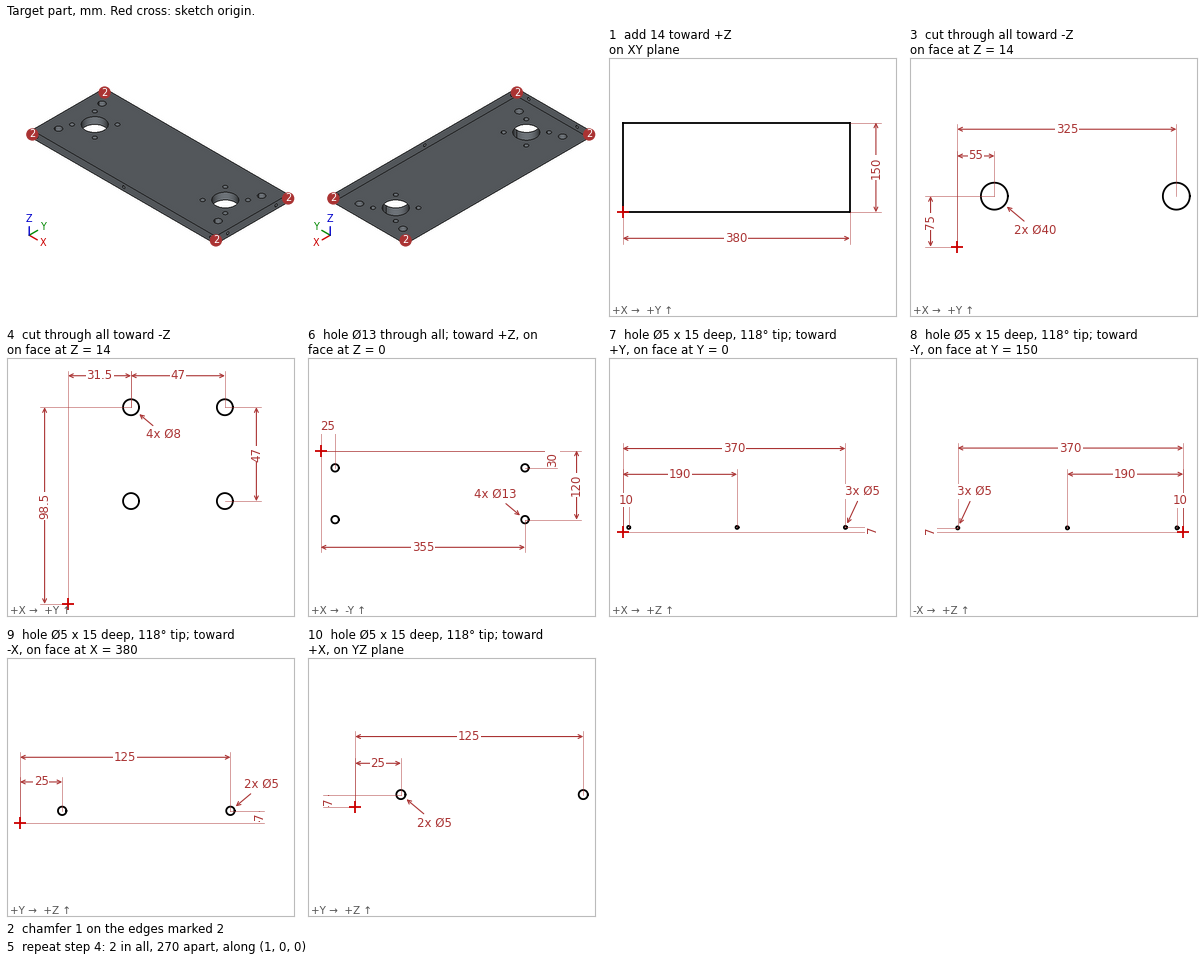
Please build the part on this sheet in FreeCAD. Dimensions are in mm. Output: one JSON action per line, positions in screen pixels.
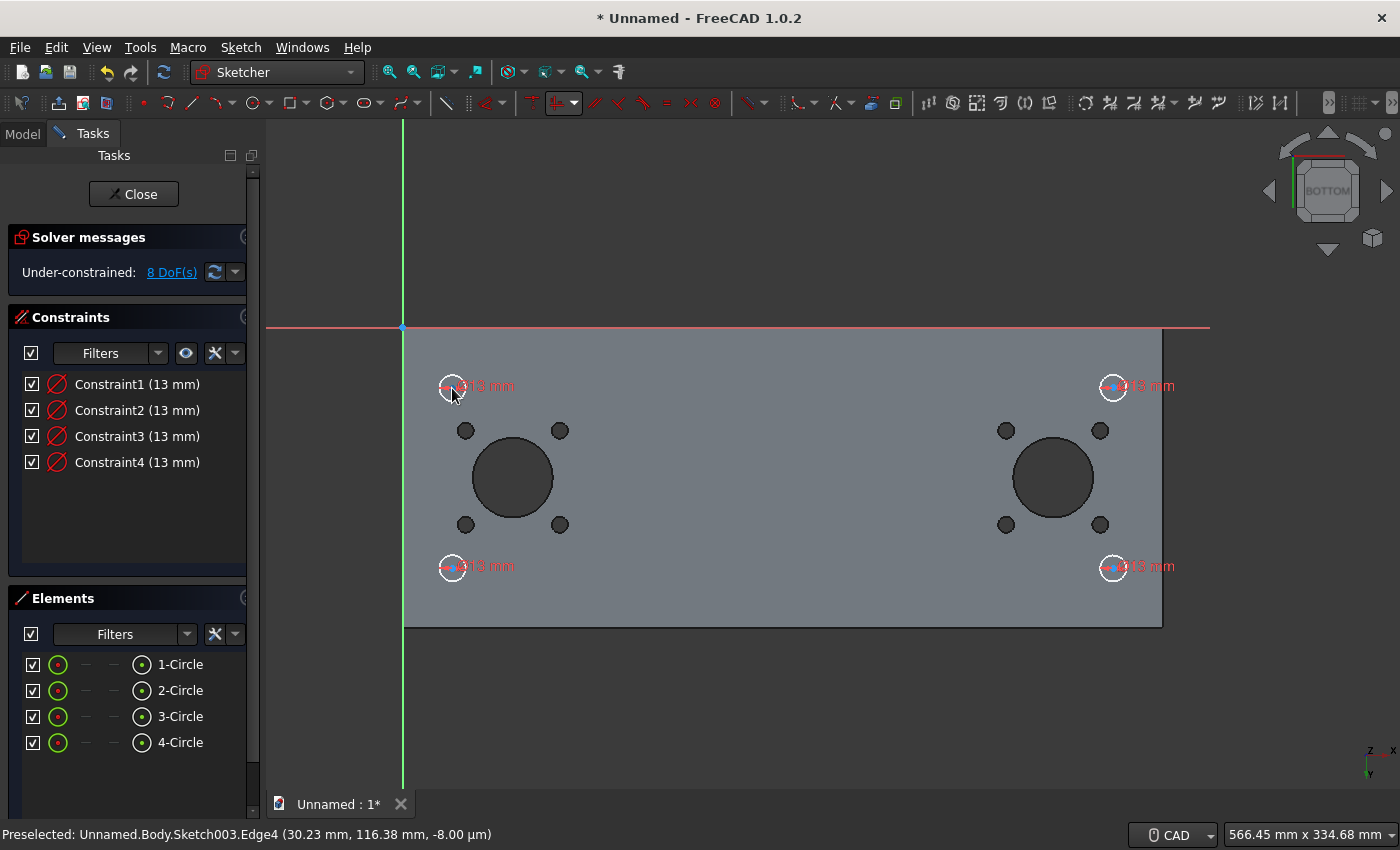
{"action": "left_click", "coordinate": [1113, 568]}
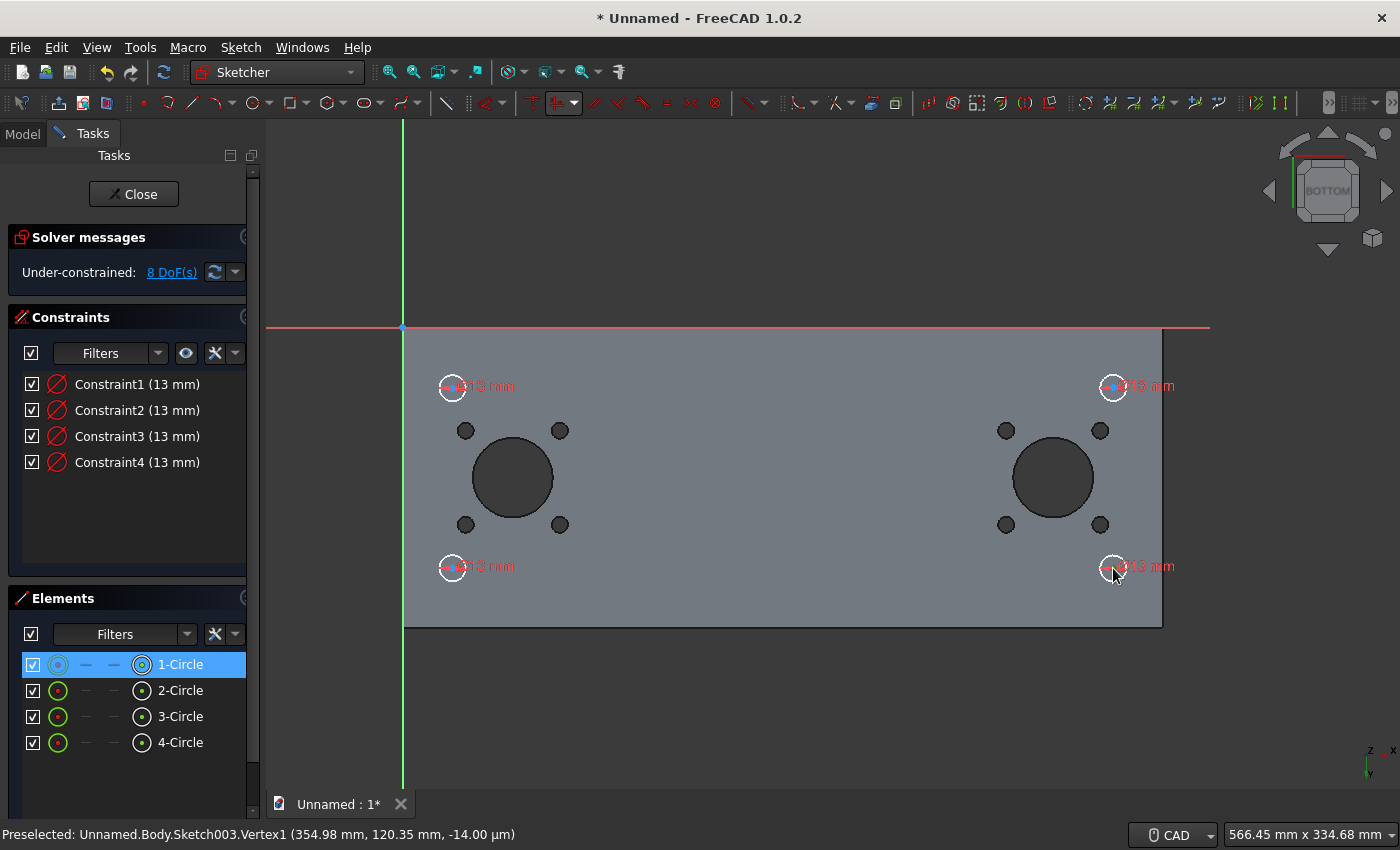
{"action": "left_click", "coordinate": [1113, 388]}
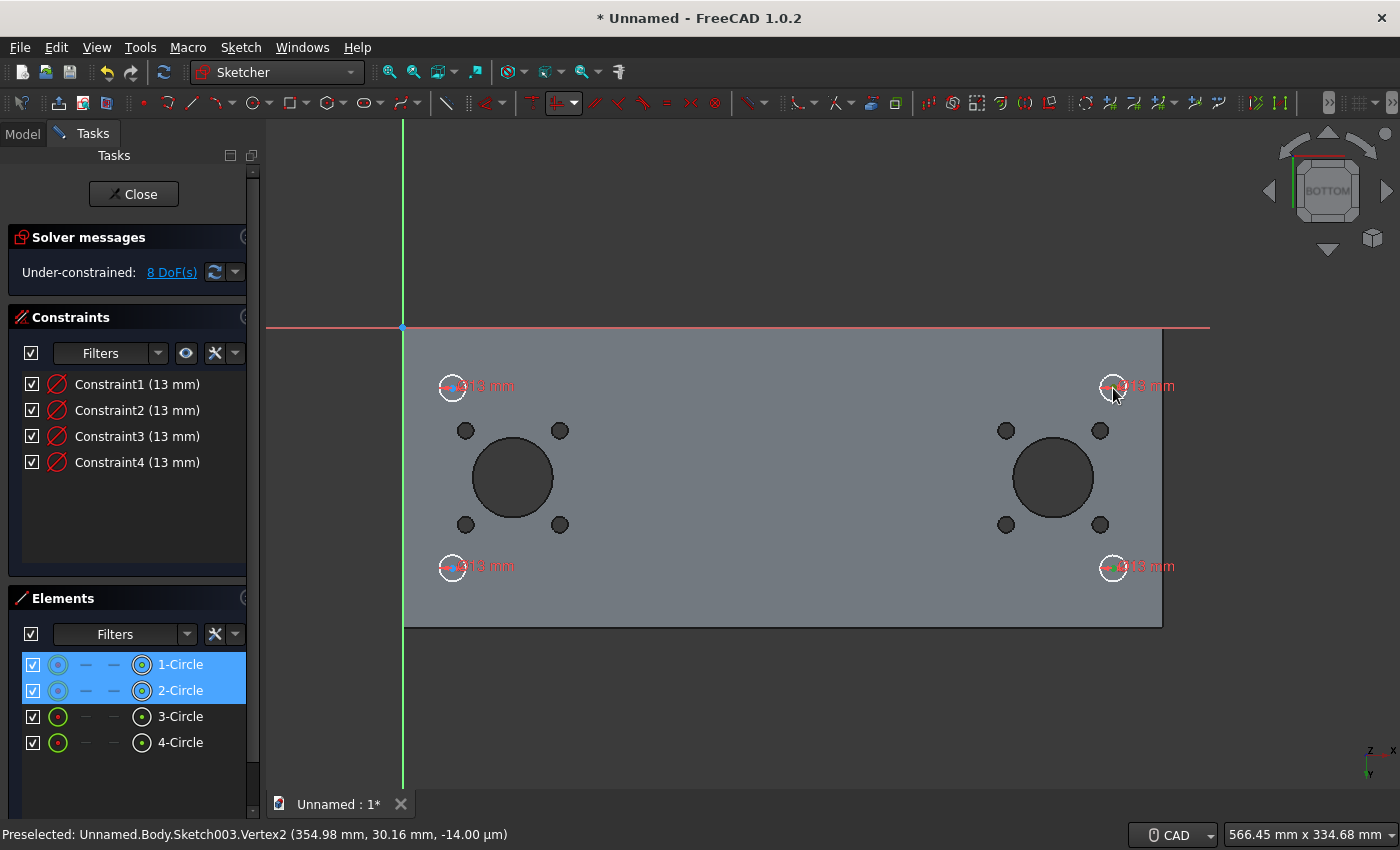
{"action": "left_click", "coordinate": [576, 104]}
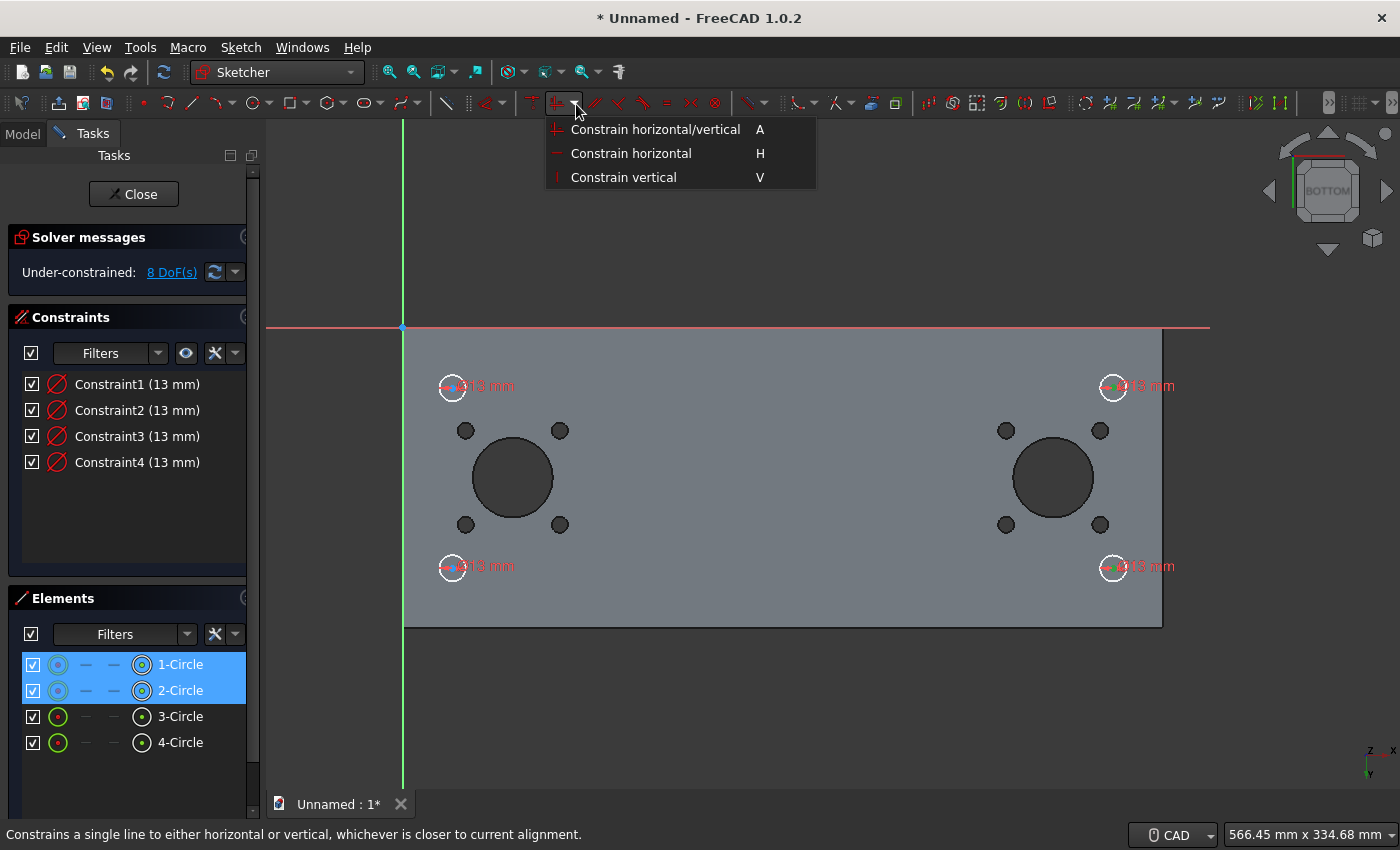
{"action": "left_click", "coordinate": [681, 177]}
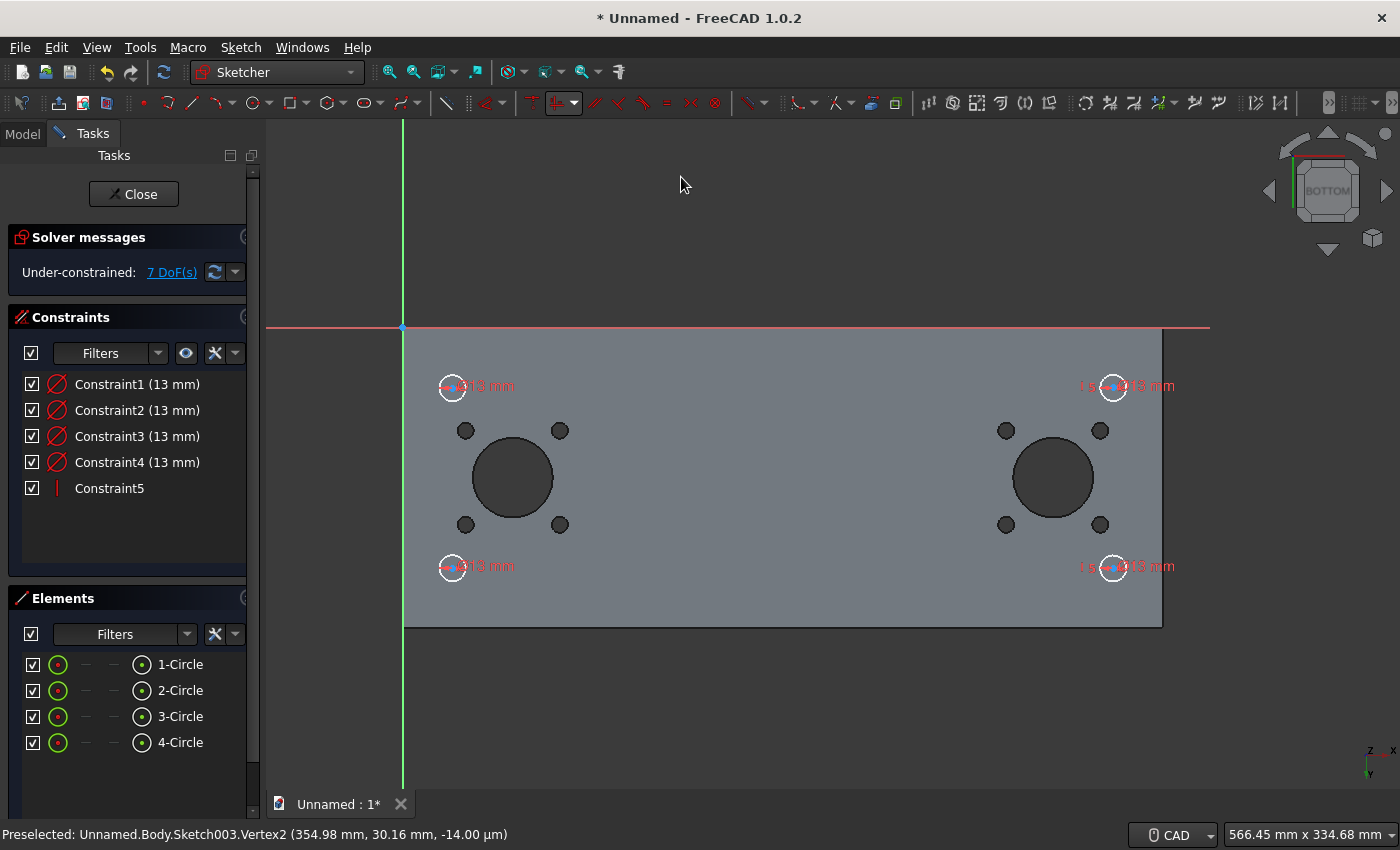
{"action": "left_click", "coordinate": [1113, 388]}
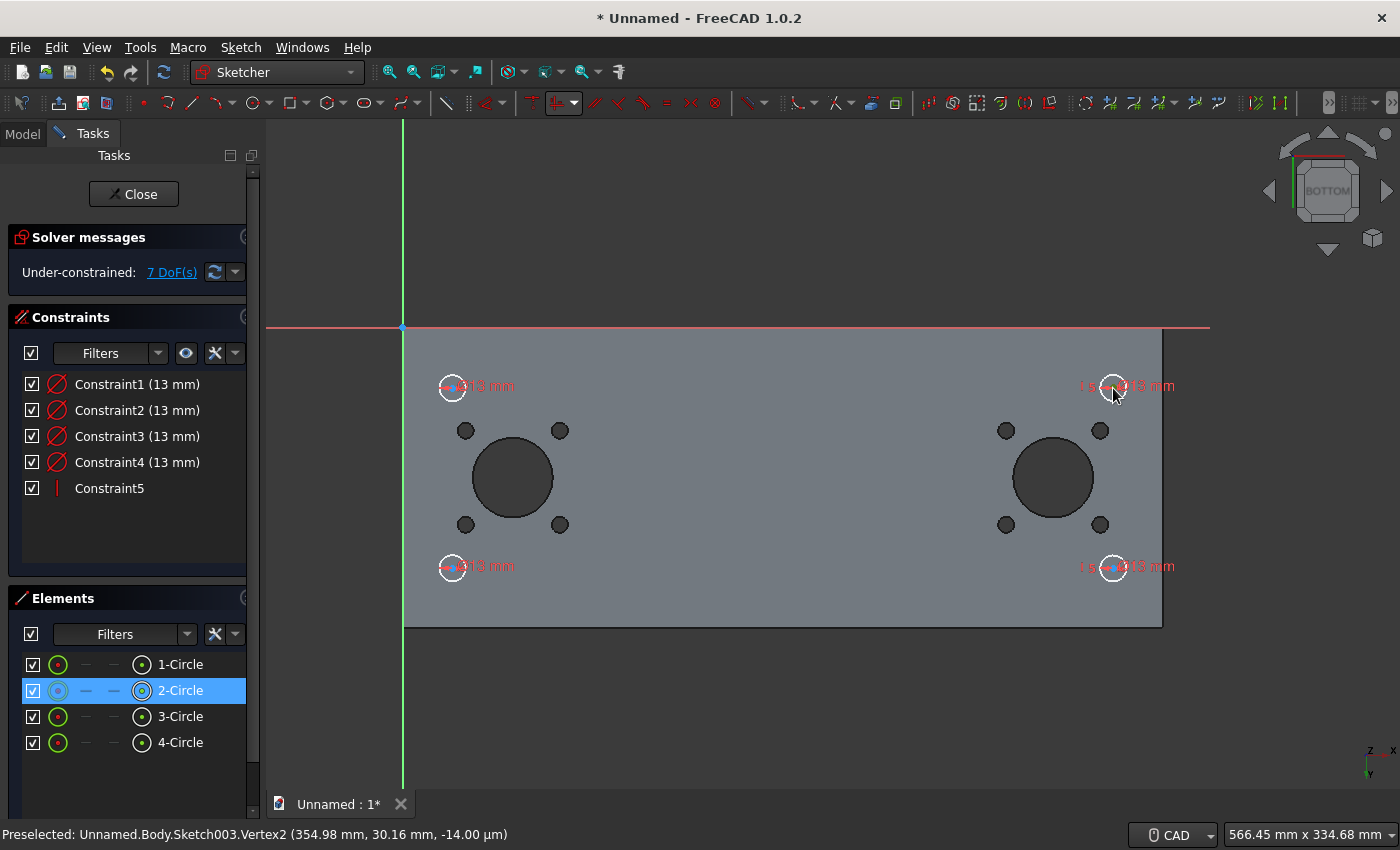
{"action": "left_click", "coordinate": [453, 388]}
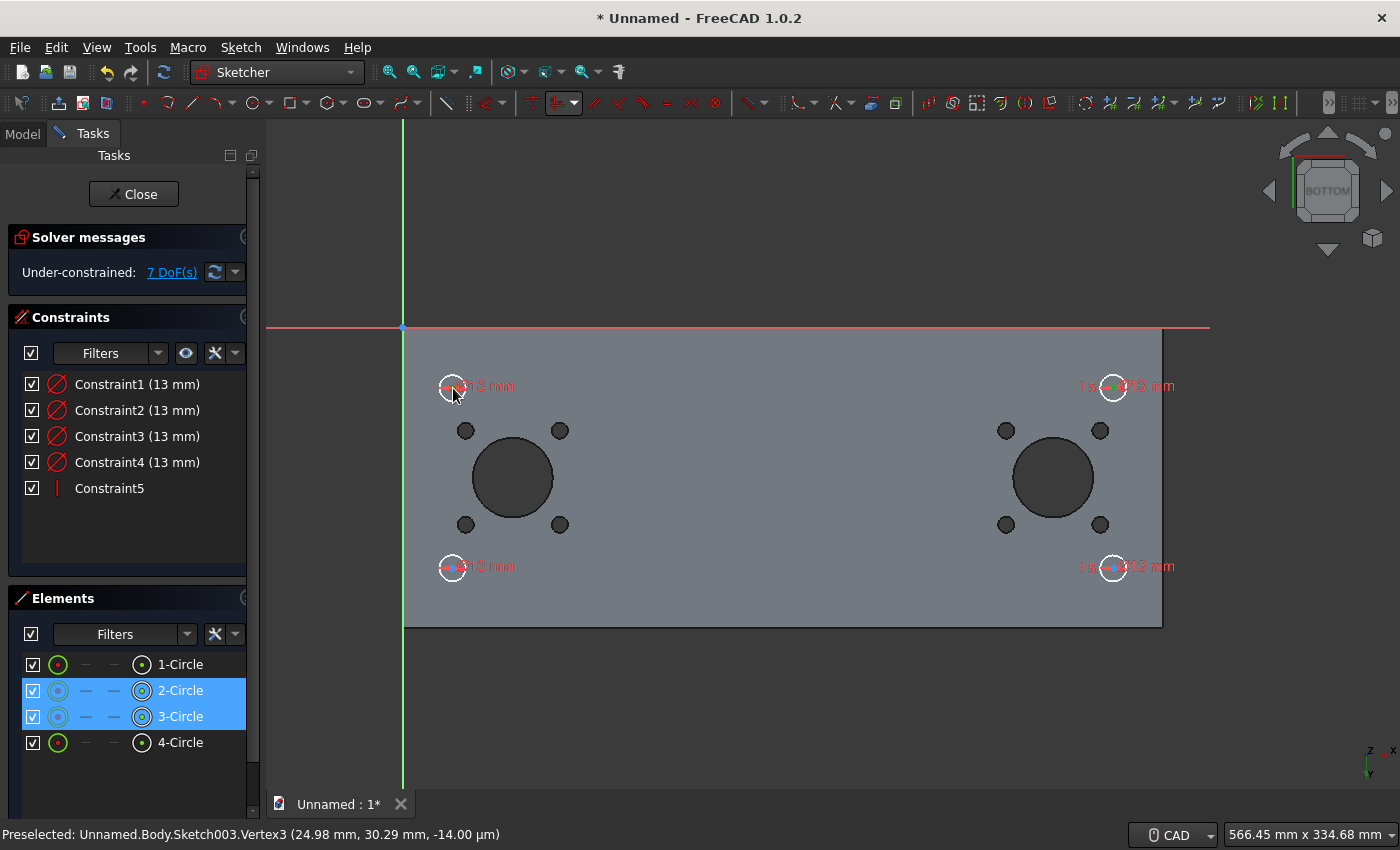
{"action": "key", "text": "h"}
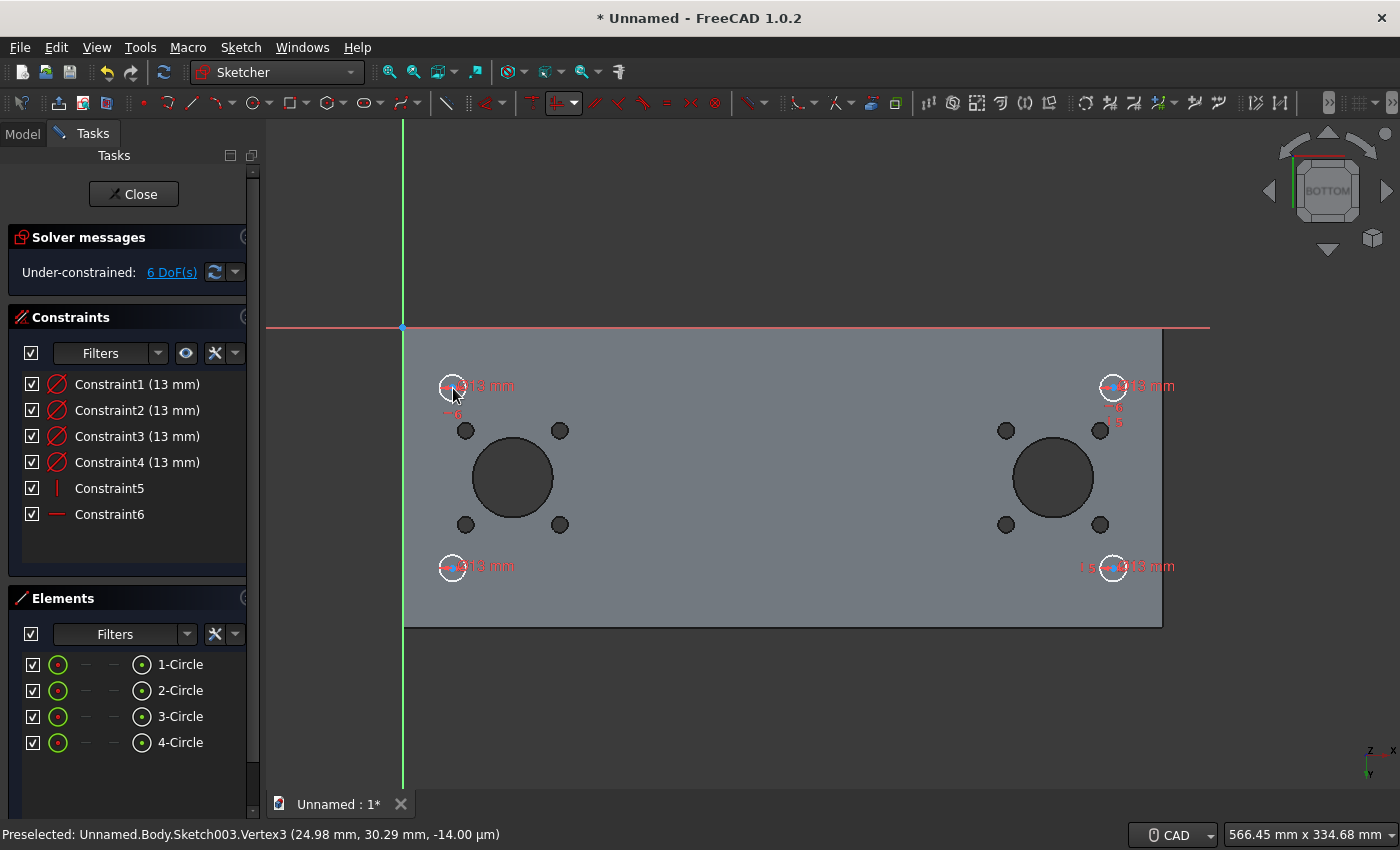
{"action": "left_click", "coordinate": [453, 388]}